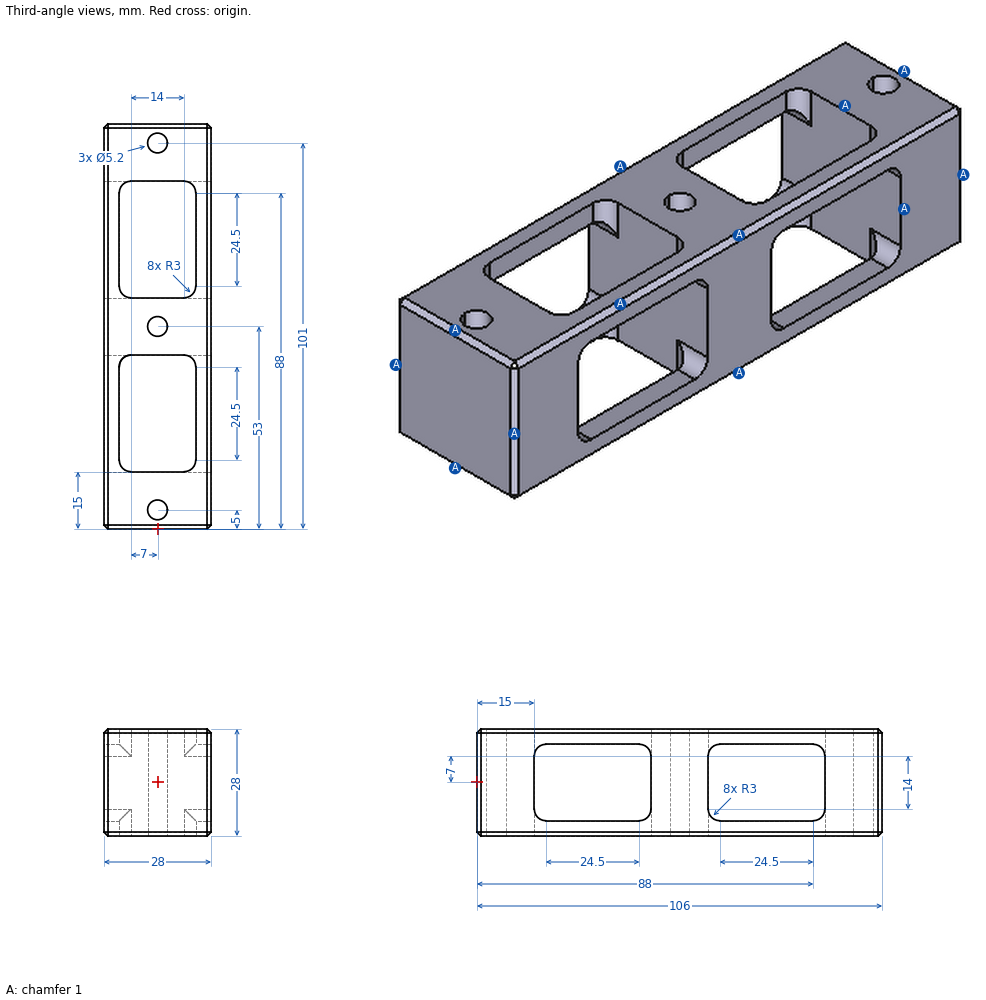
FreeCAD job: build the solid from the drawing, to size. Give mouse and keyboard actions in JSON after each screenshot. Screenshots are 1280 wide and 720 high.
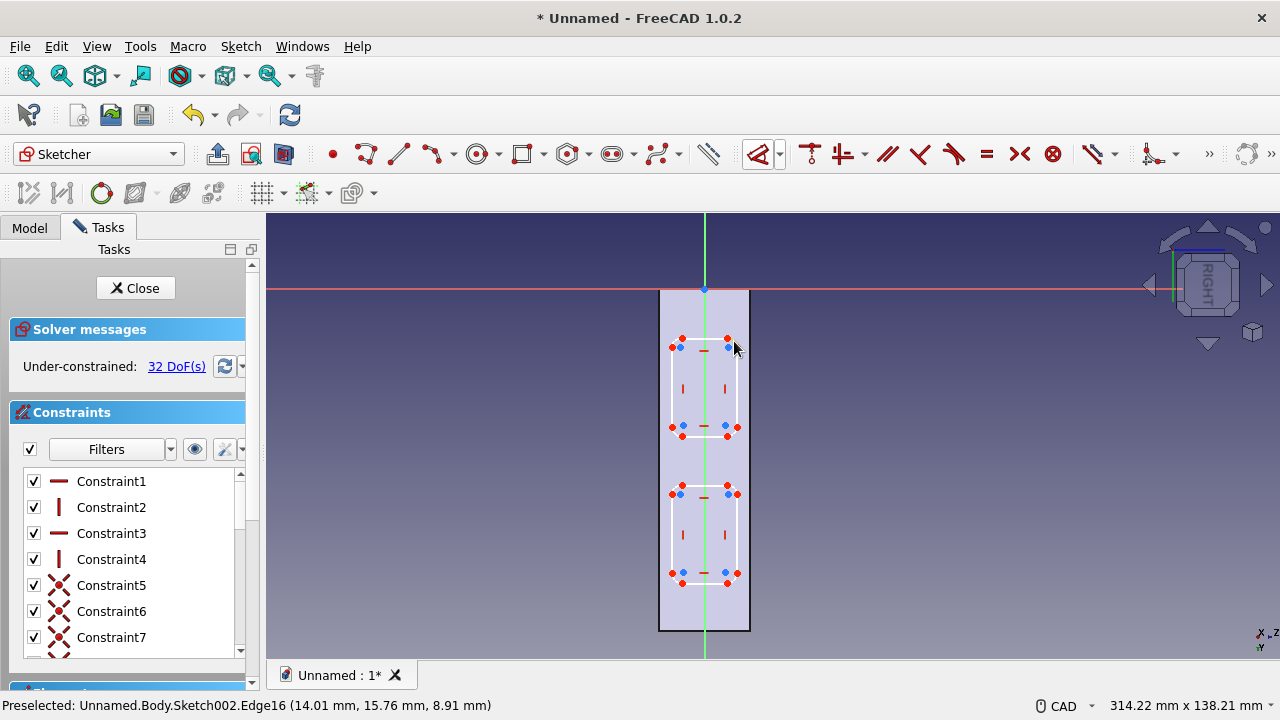
{"action": "scroll", "coordinate": [713, 486], "scroll_direction": "up", "scroll_amount": 3}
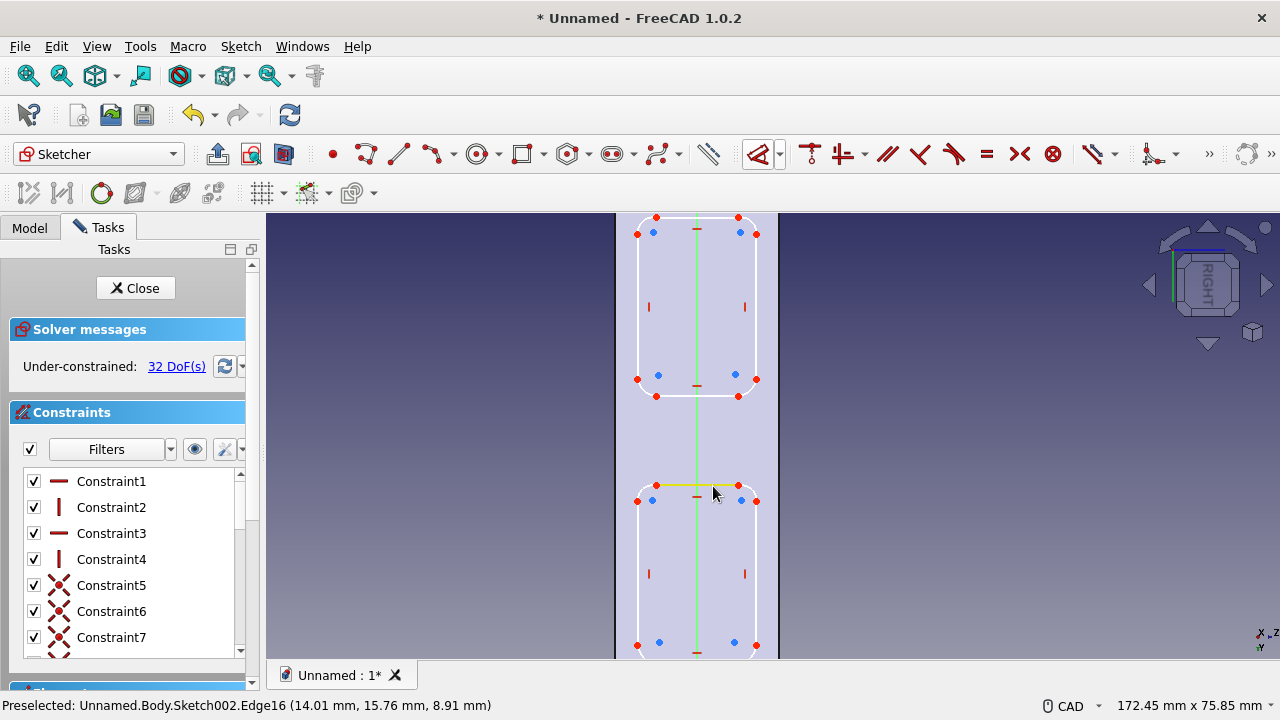
{"action": "left_click", "coordinate": [714, 485]}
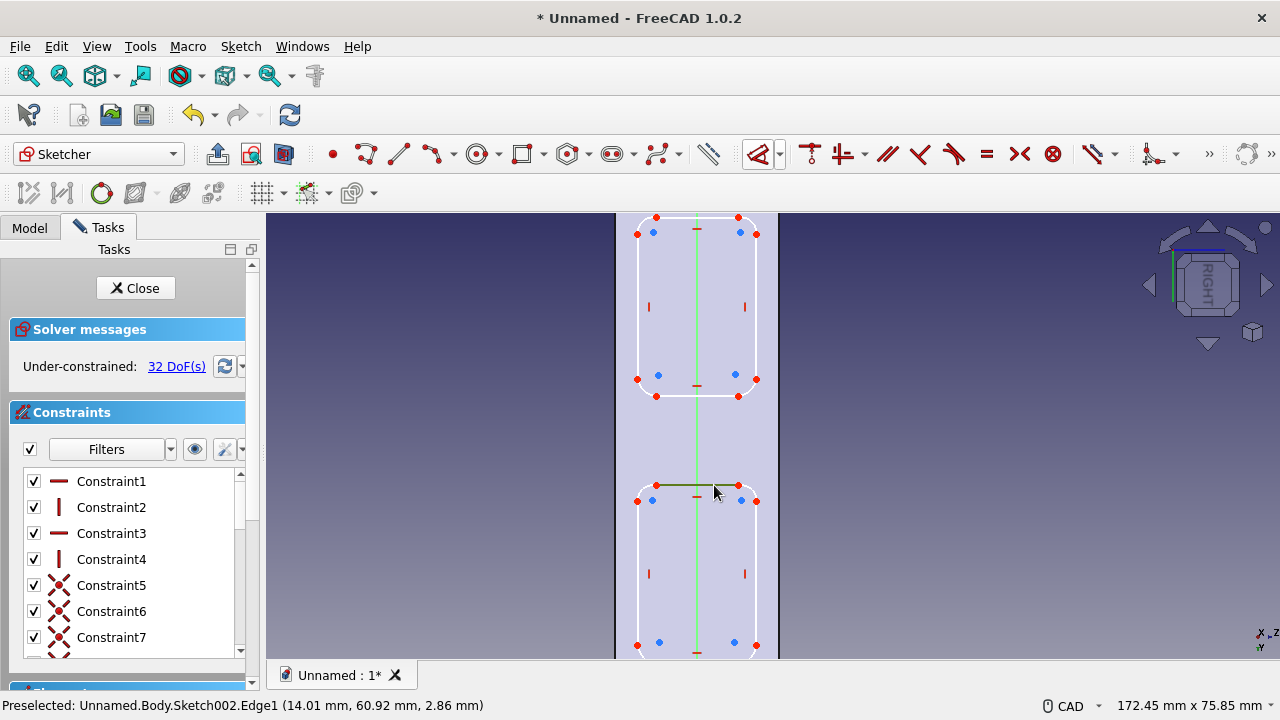
{"action": "left_click", "coordinate": [643, 489]}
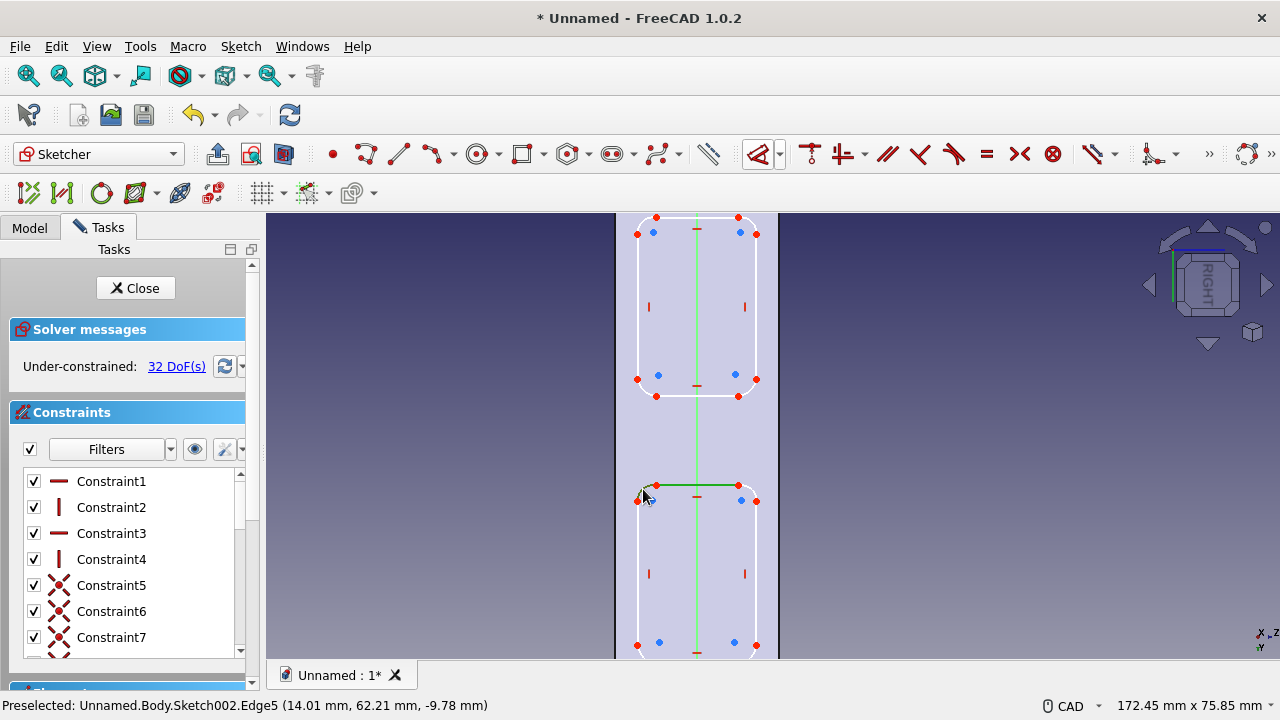
{"action": "left_click", "coordinate": [954, 154]}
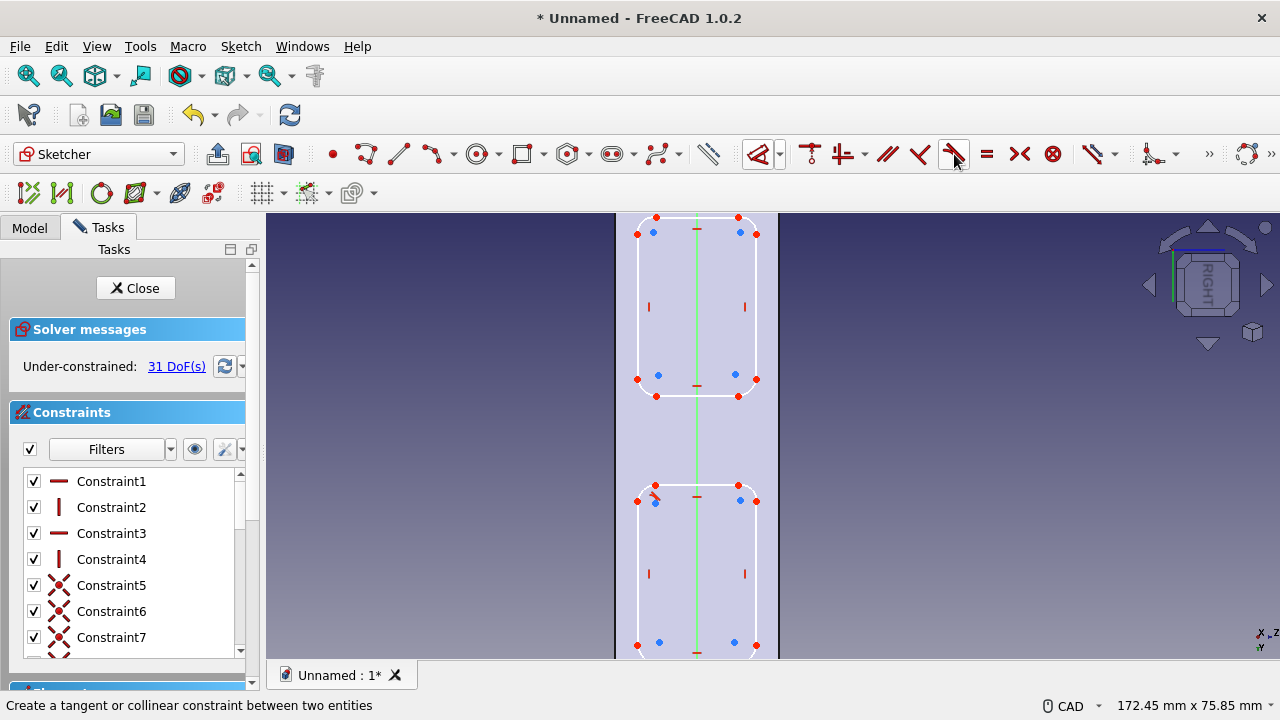
{"action": "left_click", "coordinate": [714, 485]}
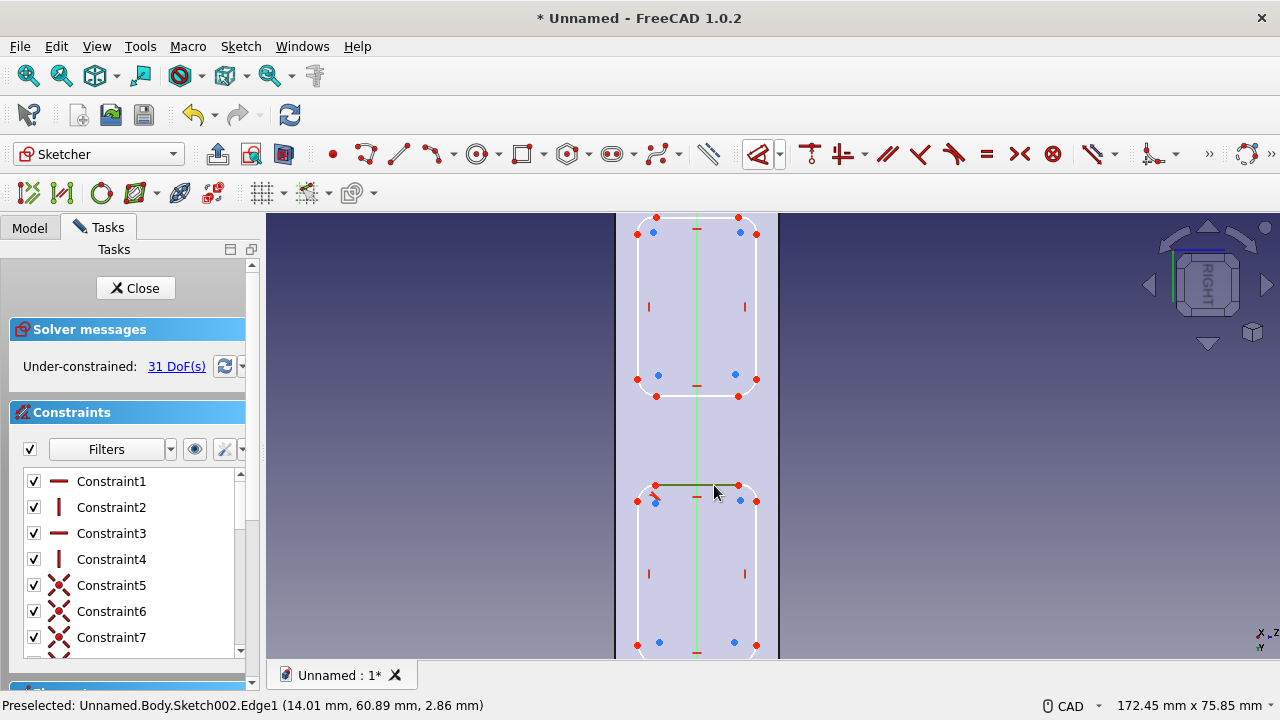
{"action": "left_click", "coordinate": [751, 489]}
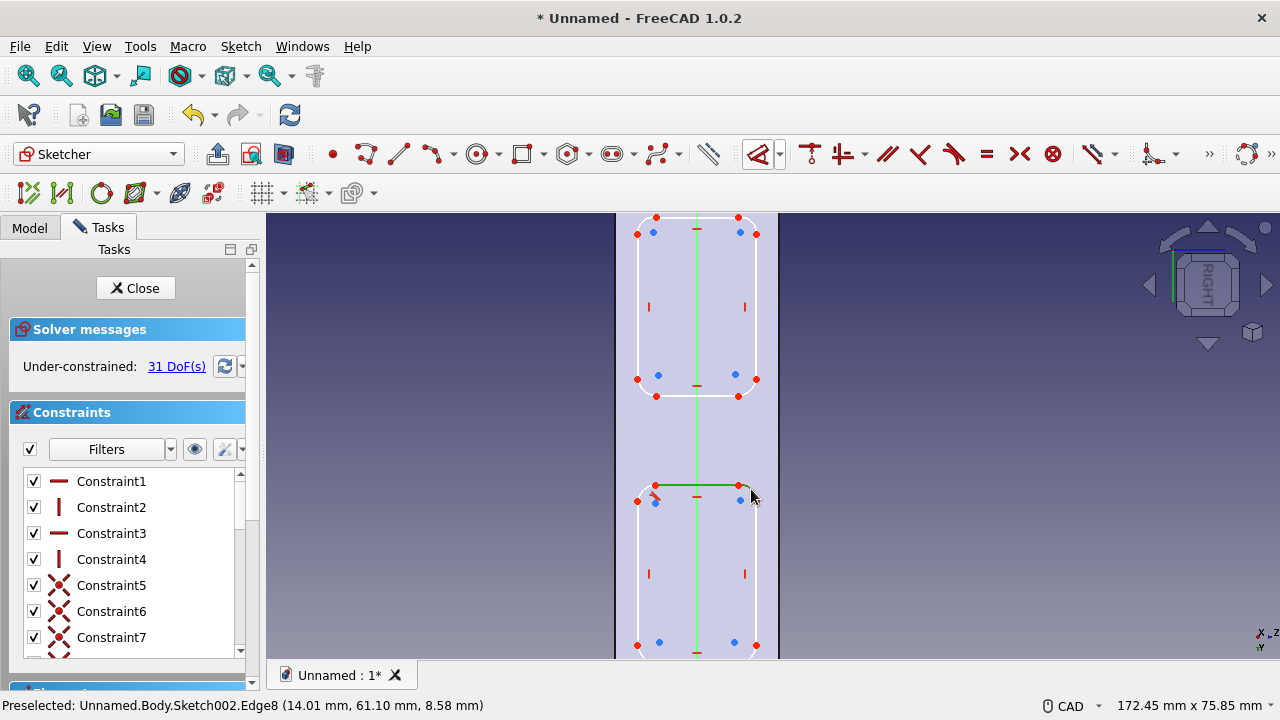
{"action": "left_click", "coordinate": [954, 154]}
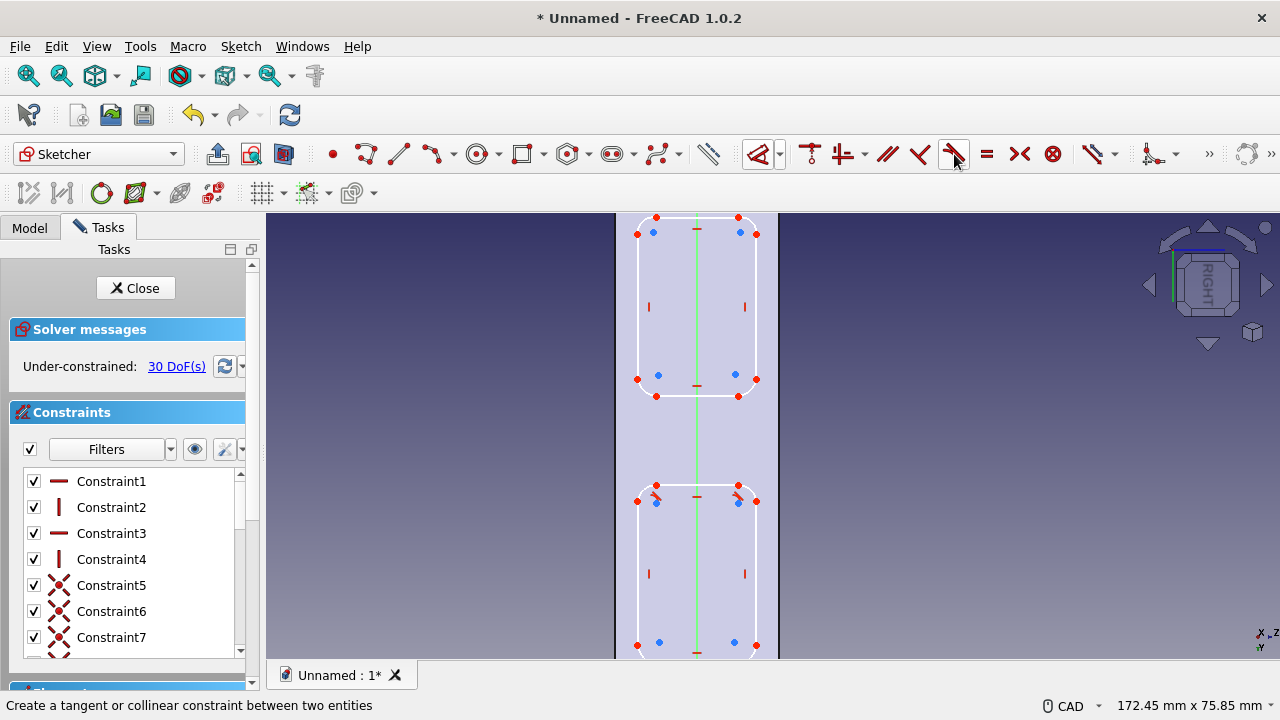
{"action": "left_click", "coordinate": [638, 545]}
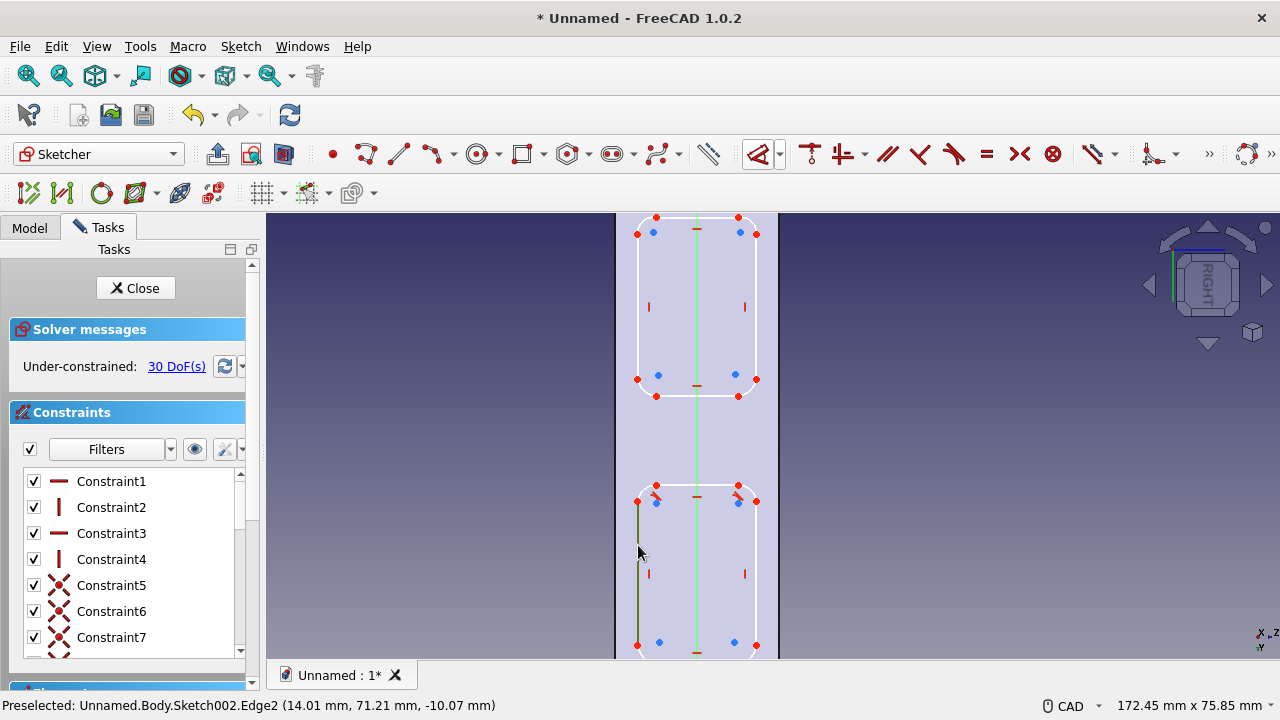
{"action": "left_click", "coordinate": [644, 490]}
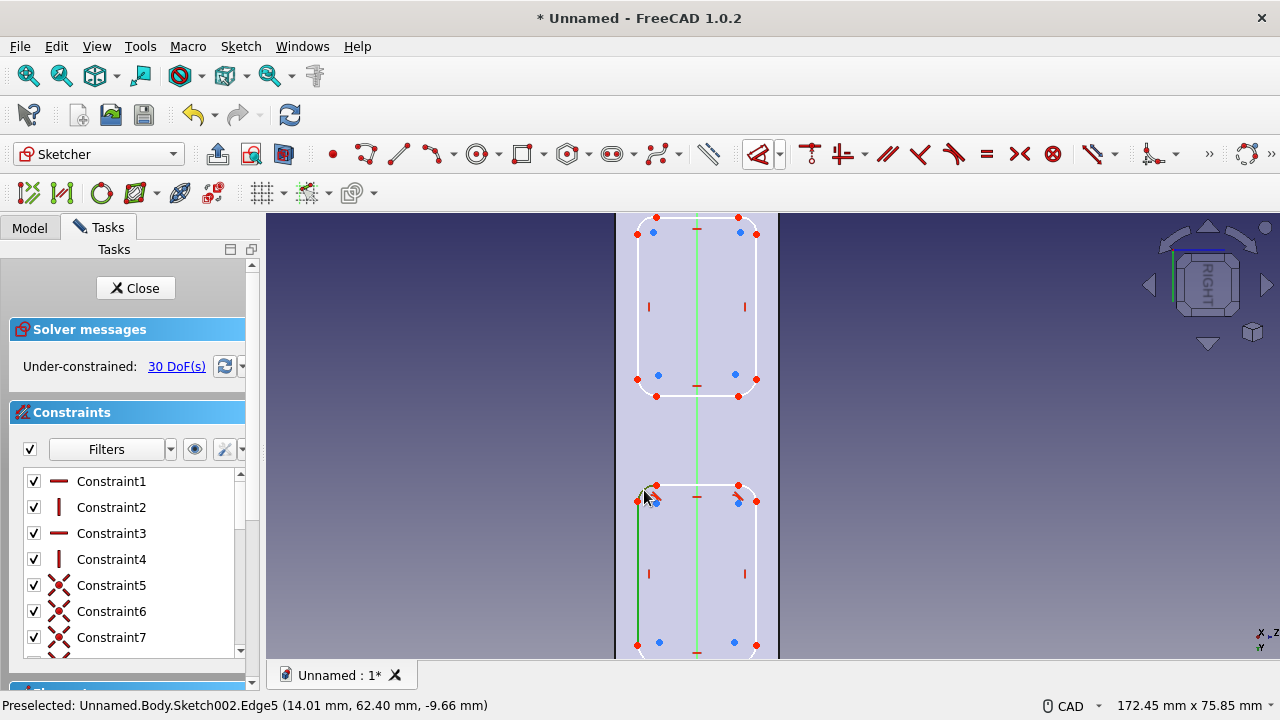
{"action": "left_click", "coordinate": [954, 154]}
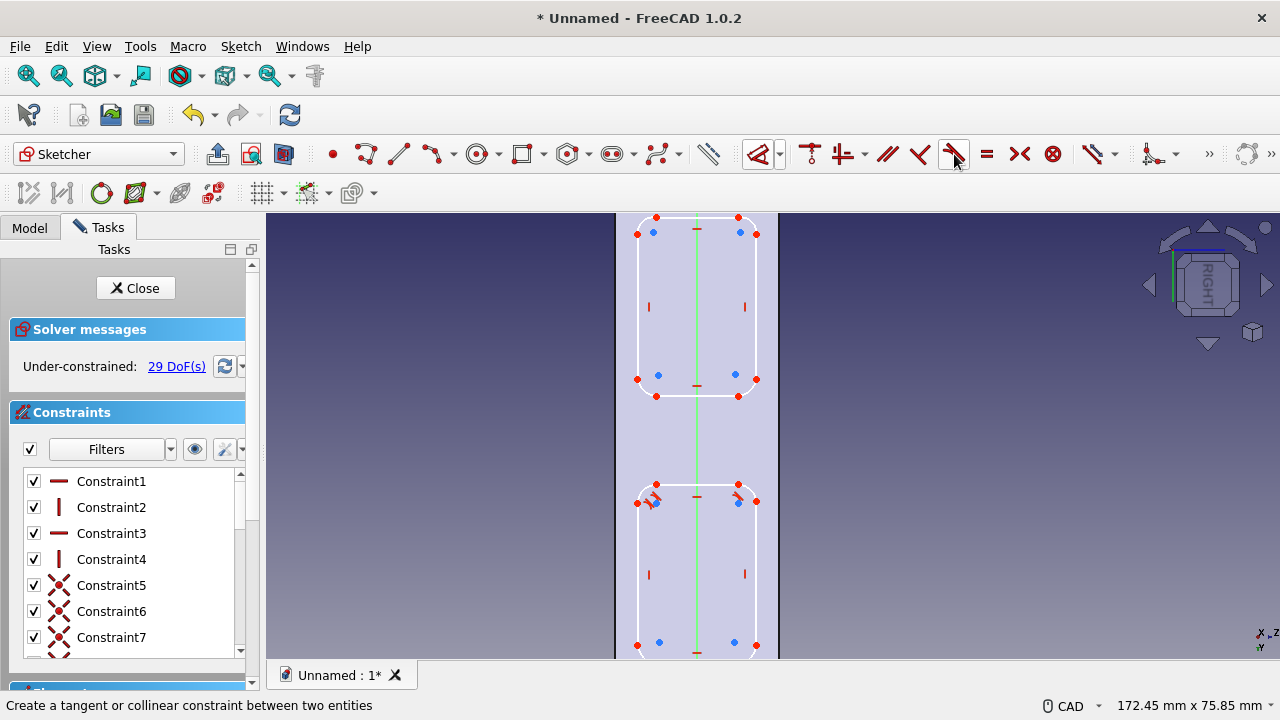
{"action": "left_click", "coordinate": [638, 546]}